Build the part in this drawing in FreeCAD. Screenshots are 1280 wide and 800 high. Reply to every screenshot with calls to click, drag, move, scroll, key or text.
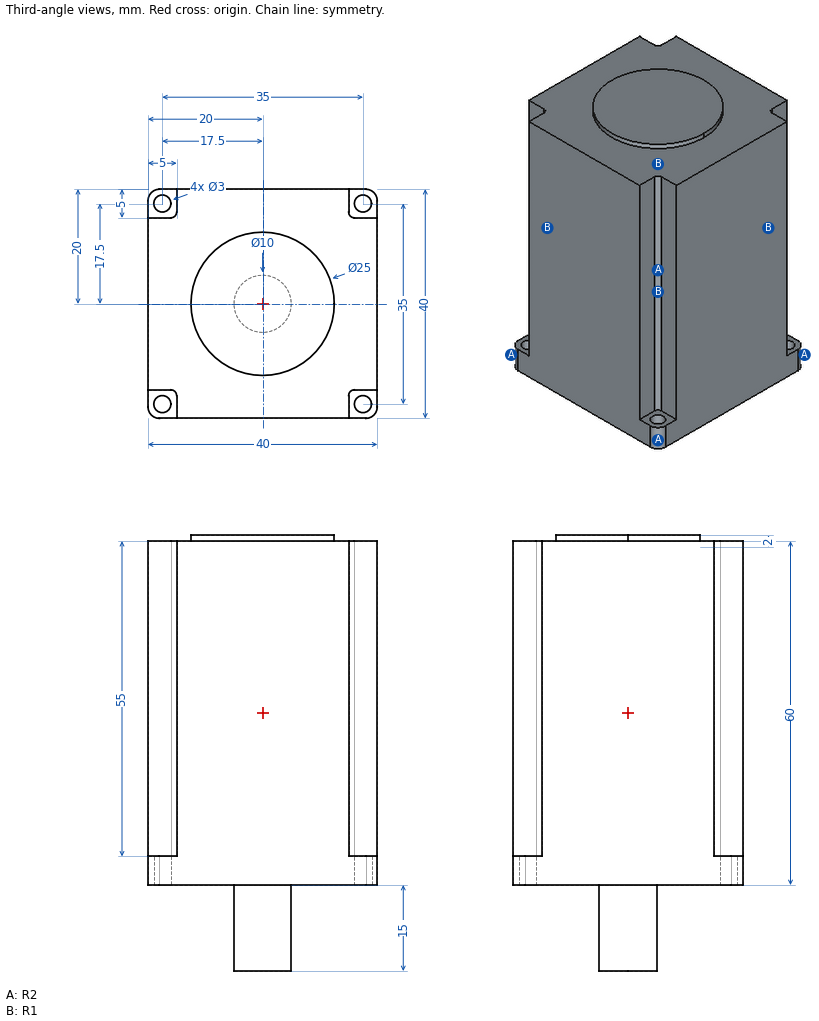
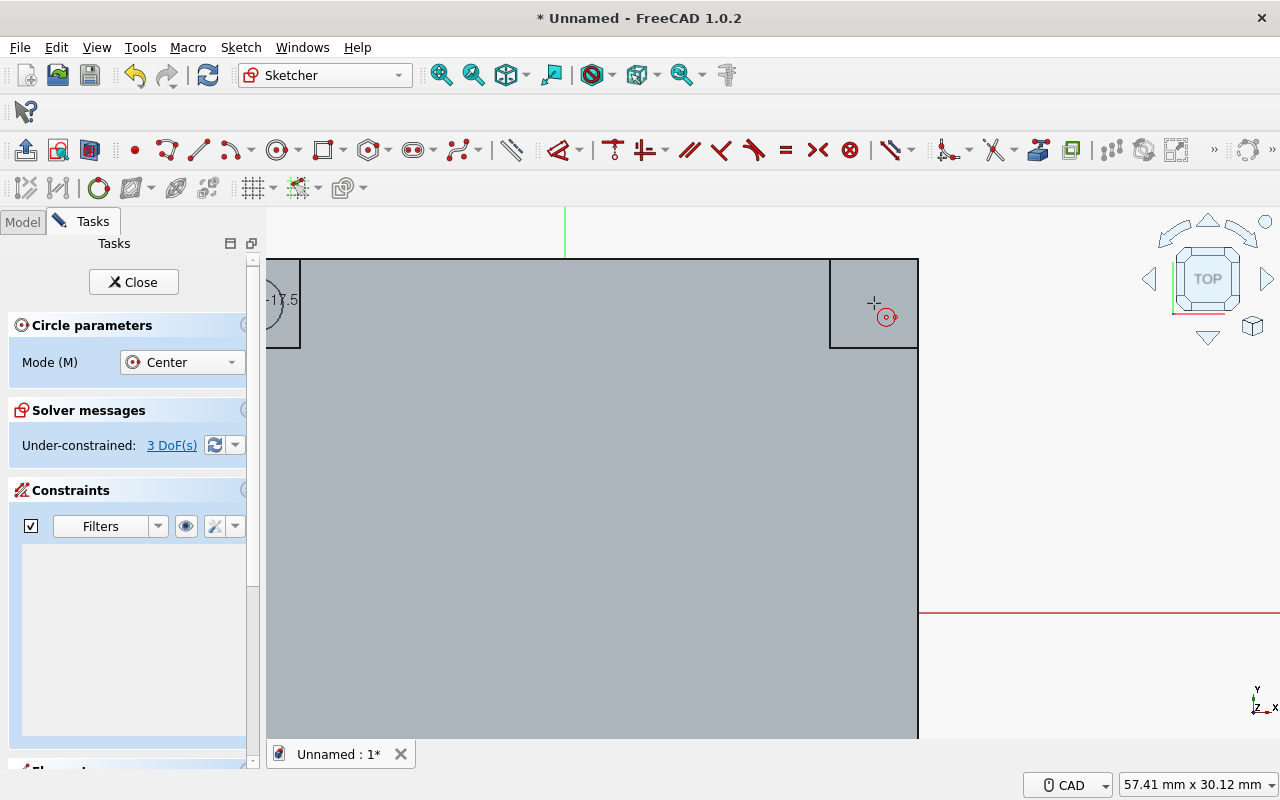
click(874, 304)
click(893, 285)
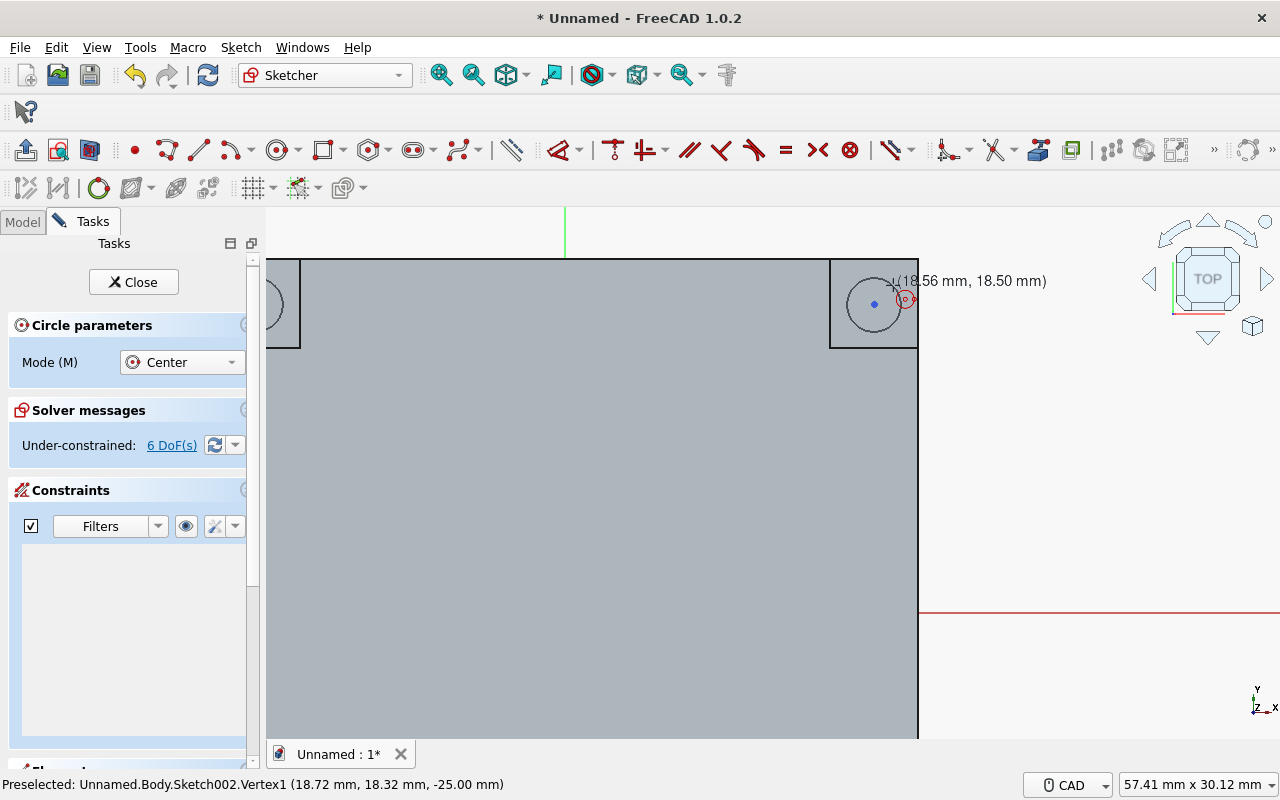
scroll(874, 303, down, 3)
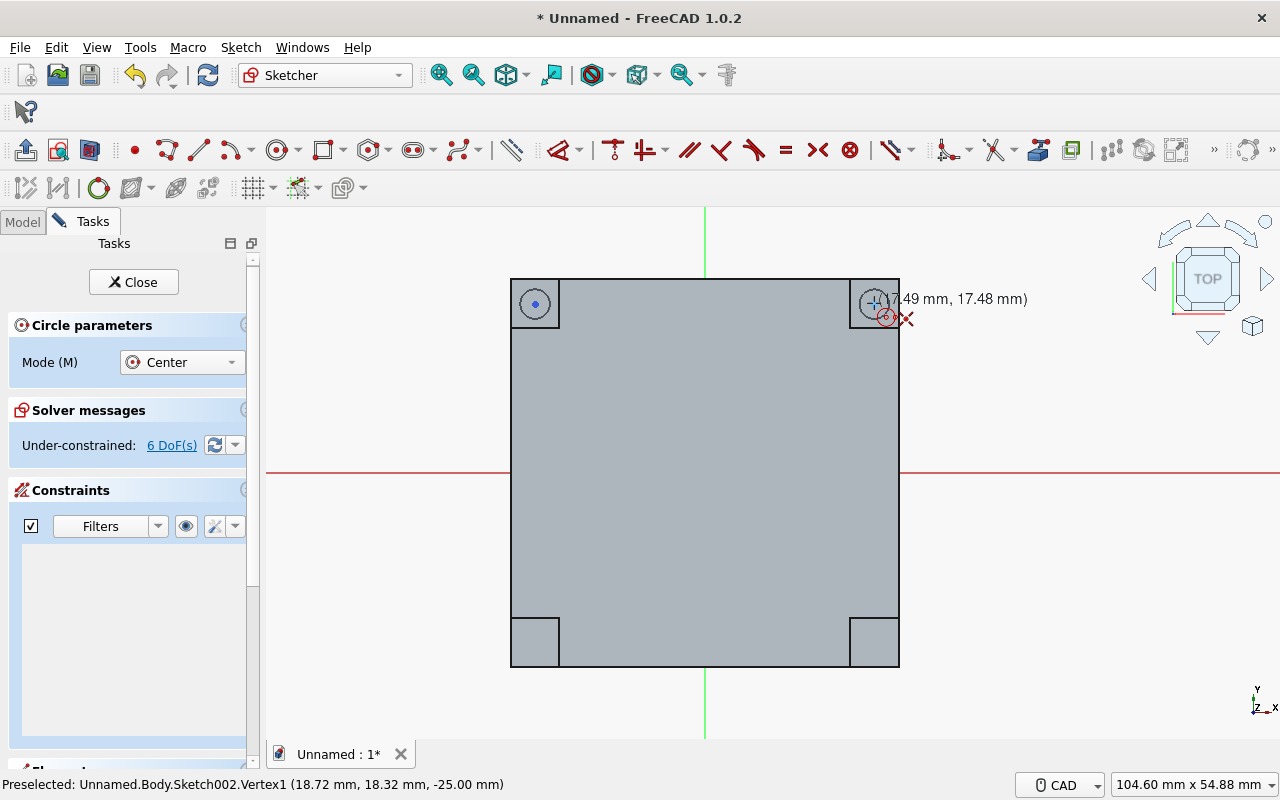
scroll(874, 643, up, 3)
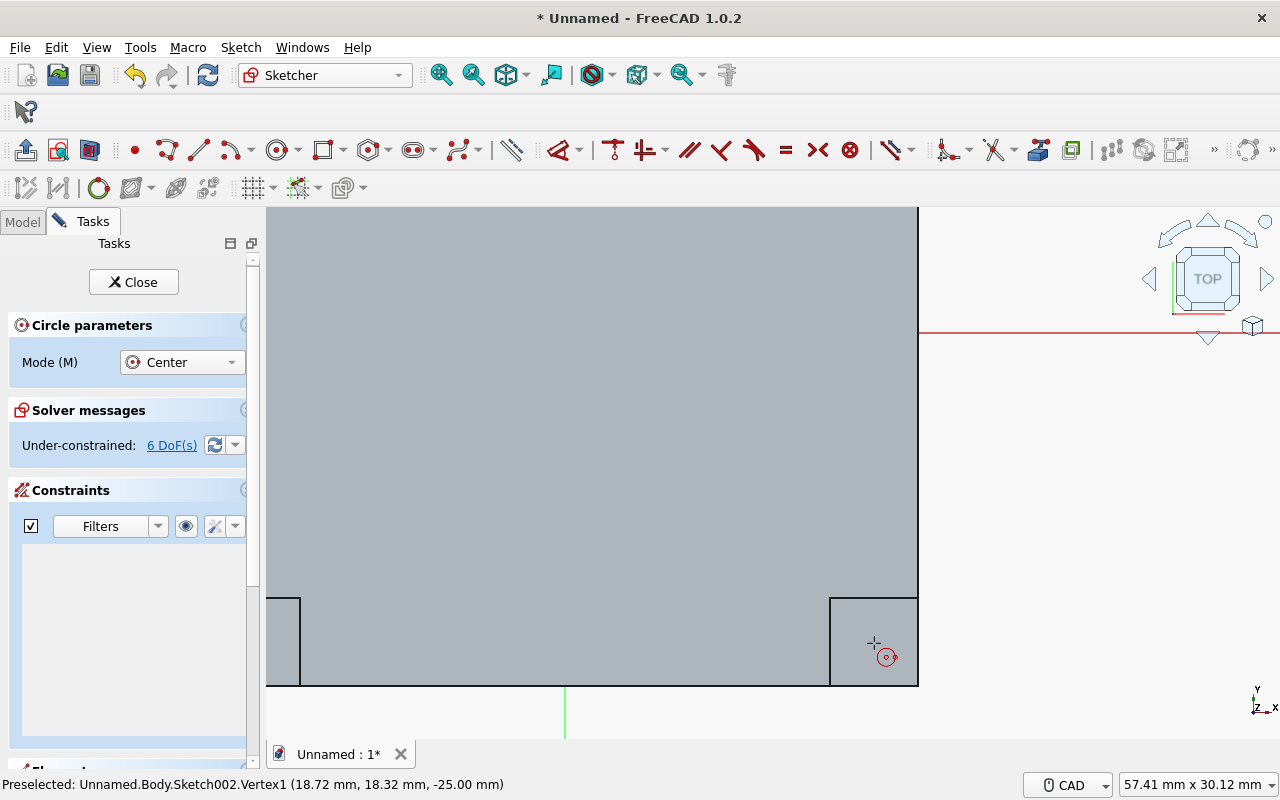
click(874, 642)
click(893, 623)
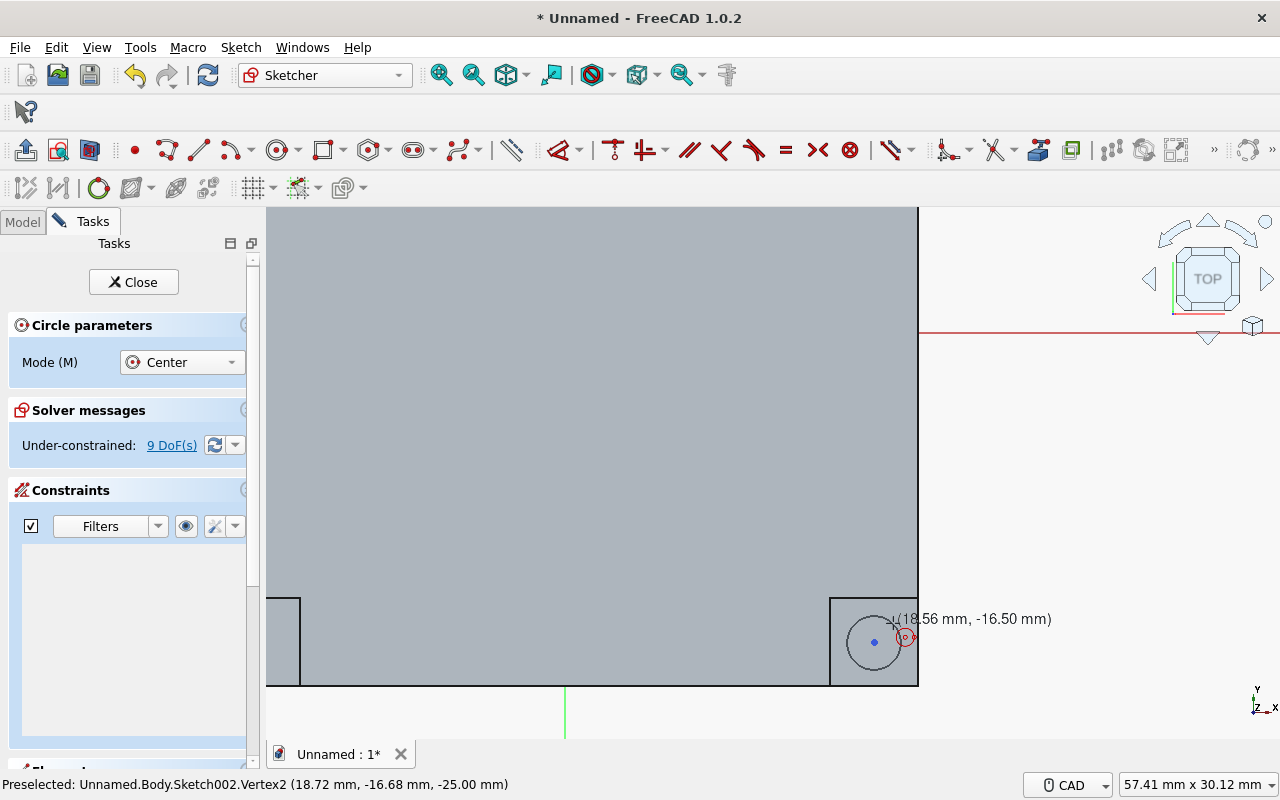
scroll(874, 644, down, 3)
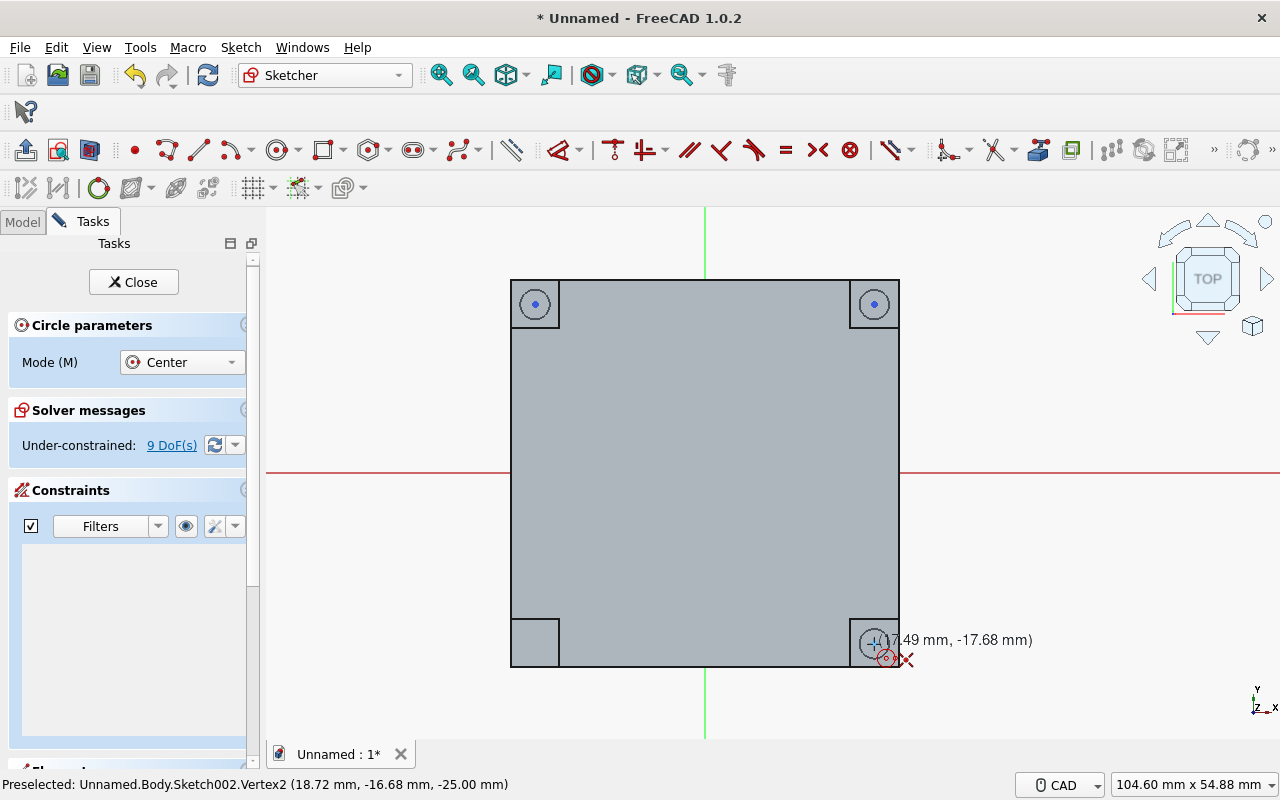
scroll(535, 643, up, 3)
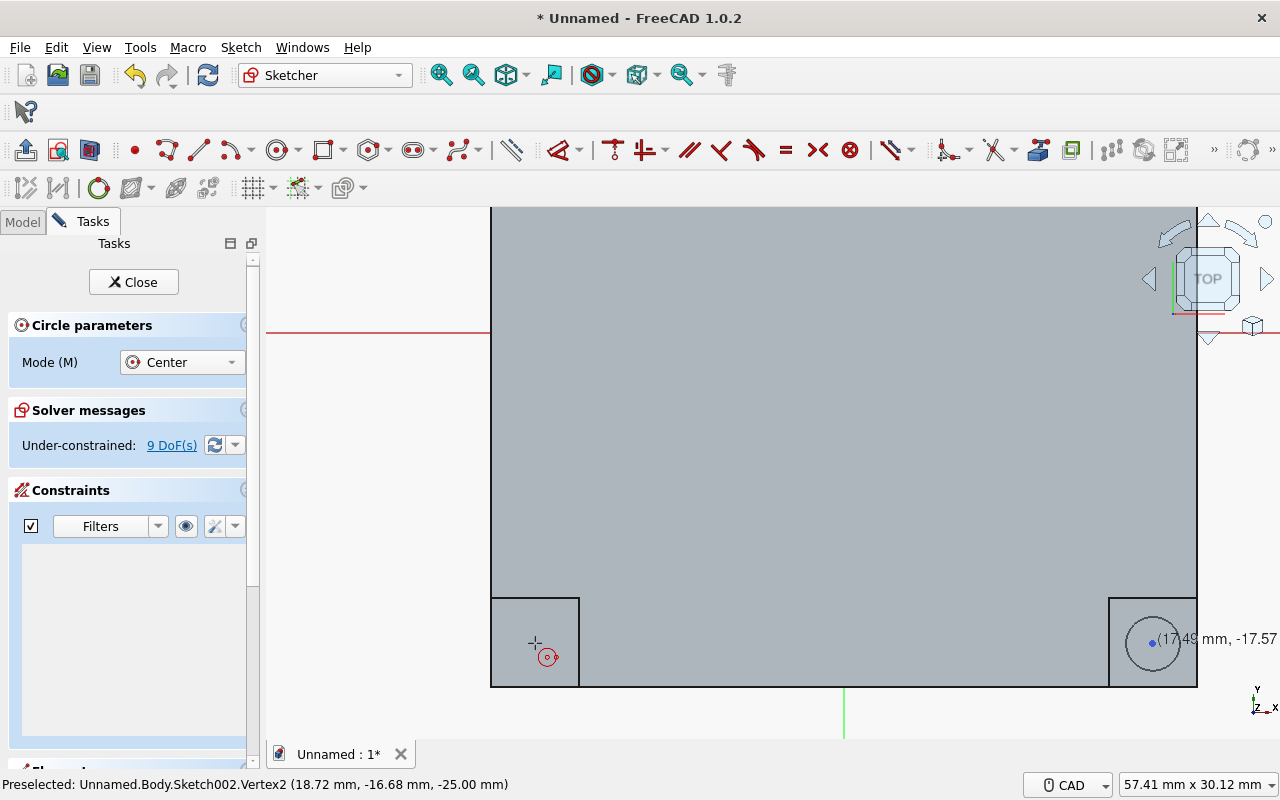
click(535, 643)
click(554, 624)
key(Escape)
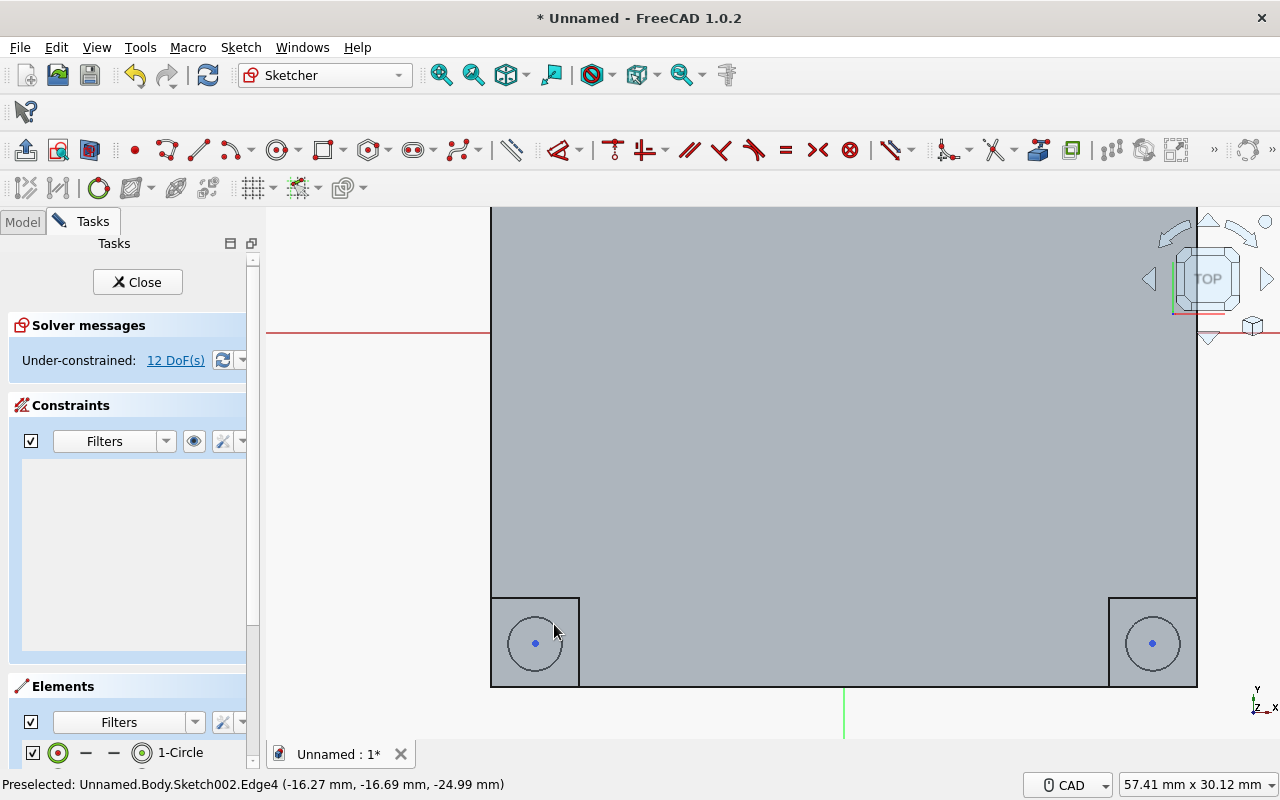
scroll(535, 643, down, 3)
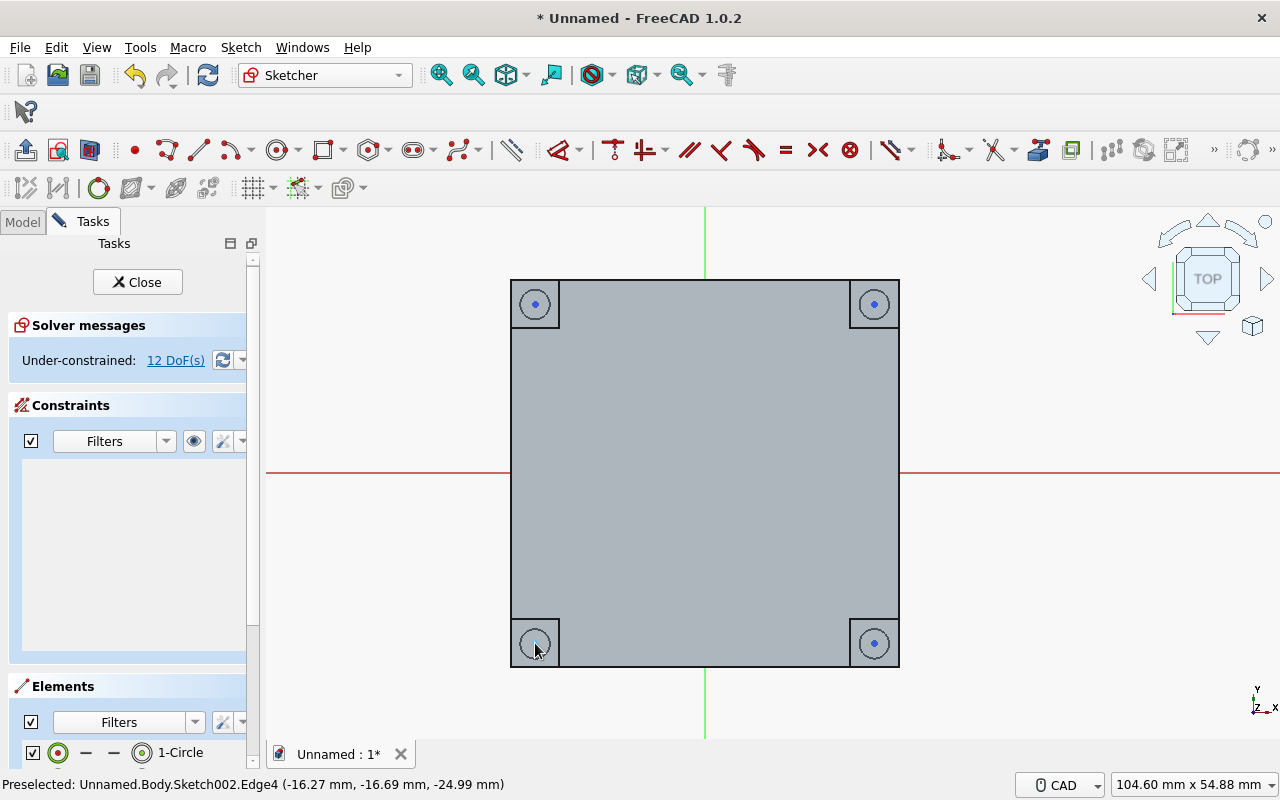
click(545, 294)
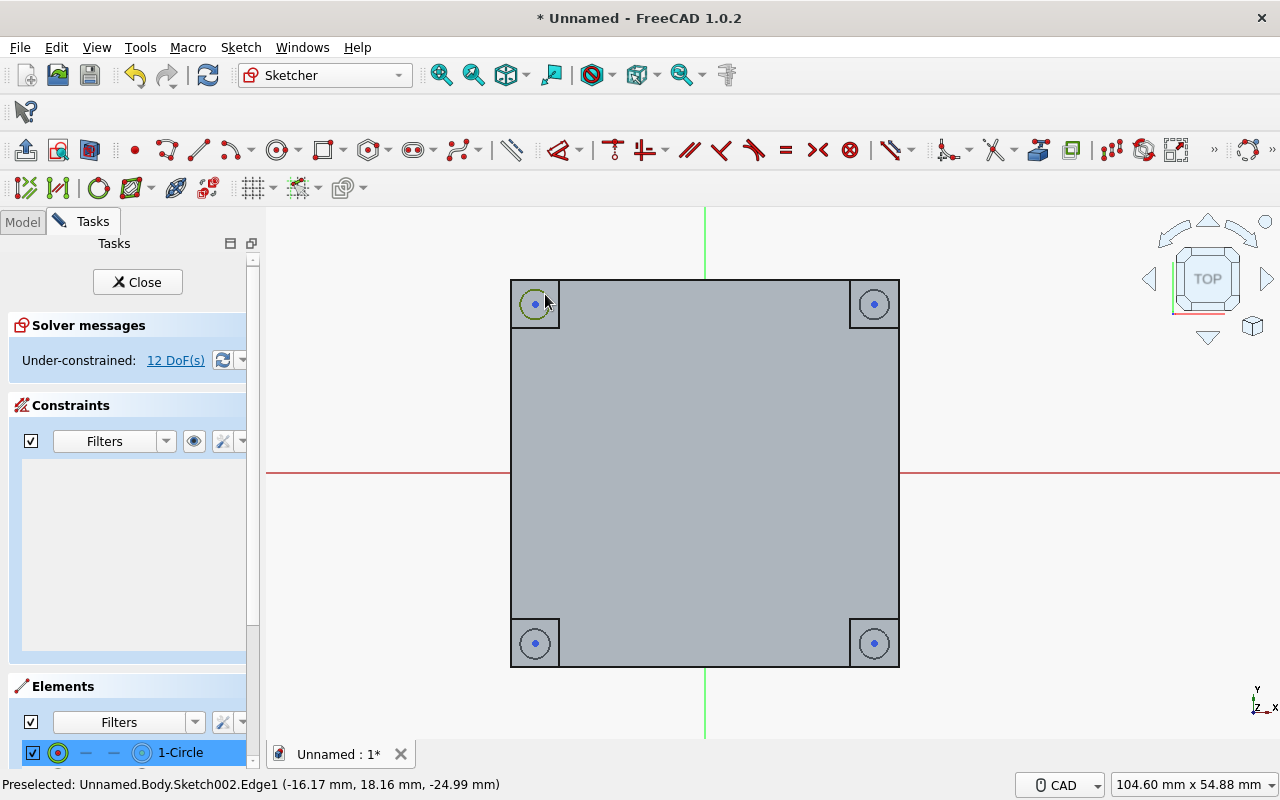
click(885, 294)